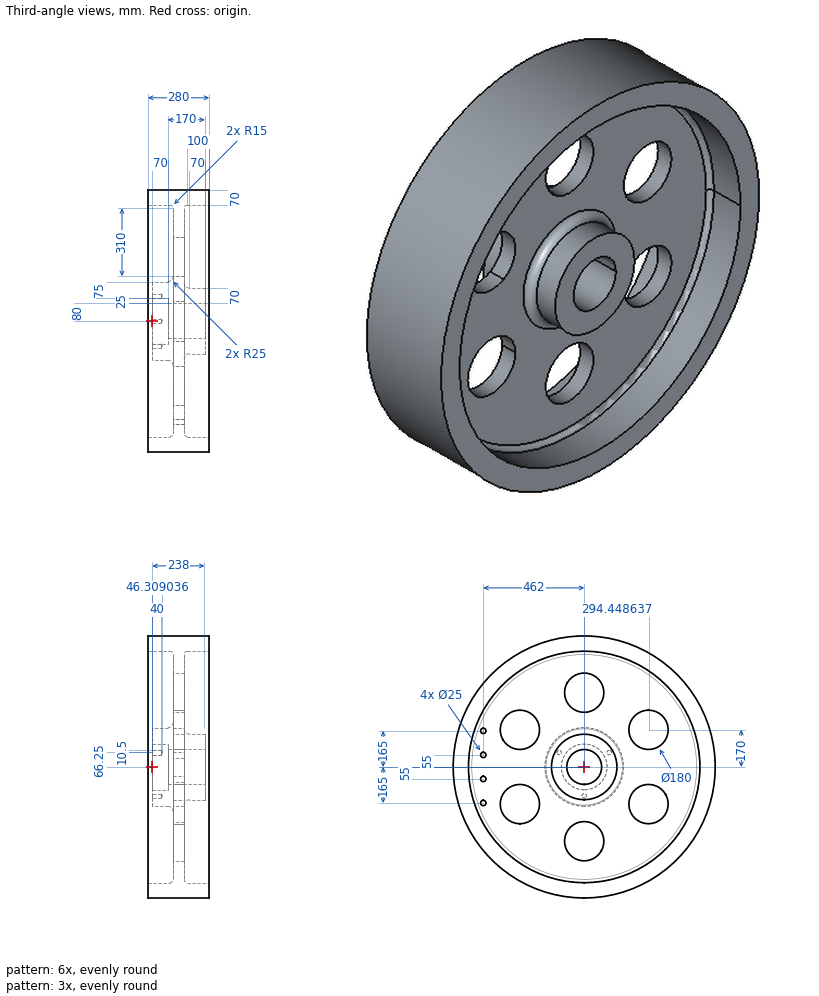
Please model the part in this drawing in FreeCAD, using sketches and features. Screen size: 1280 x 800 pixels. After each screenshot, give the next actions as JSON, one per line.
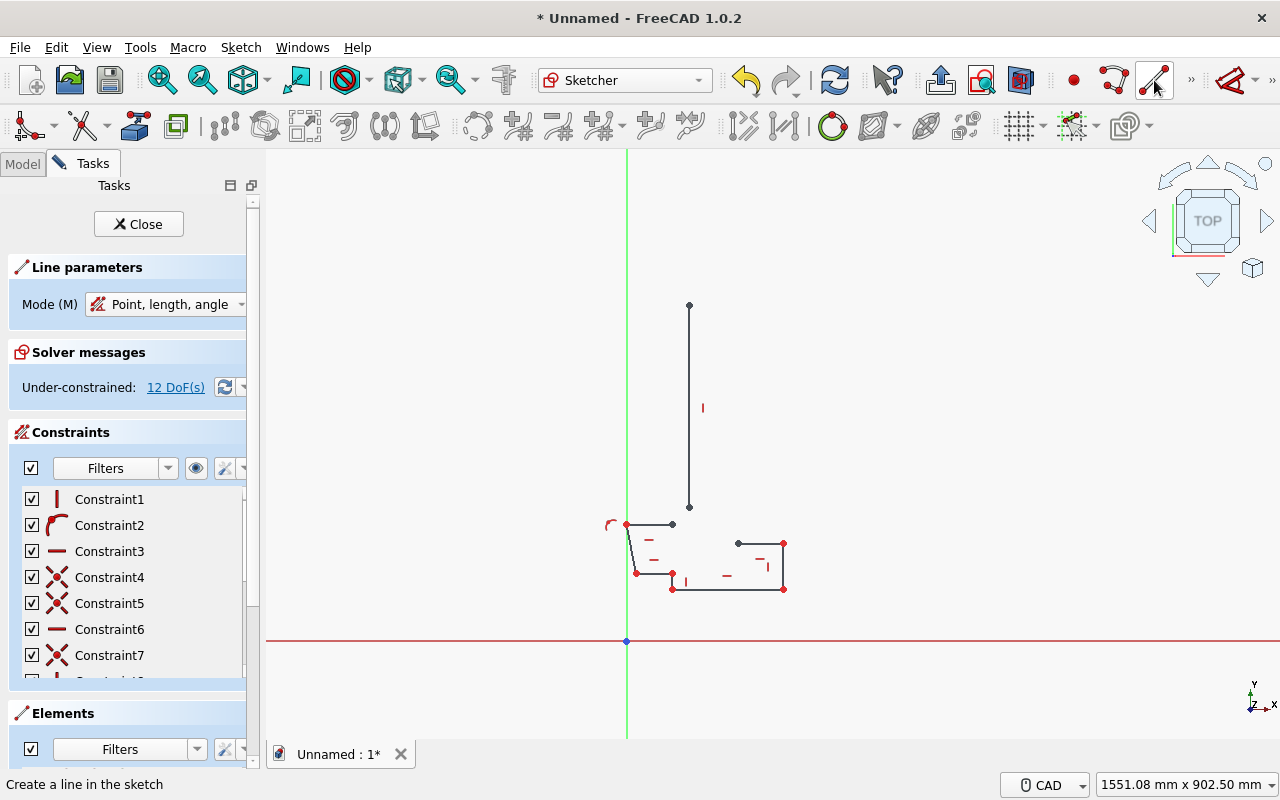
{"action": "left_click", "coordinate": [721, 527]}
{"action": "left_click", "coordinate": [721, 305]}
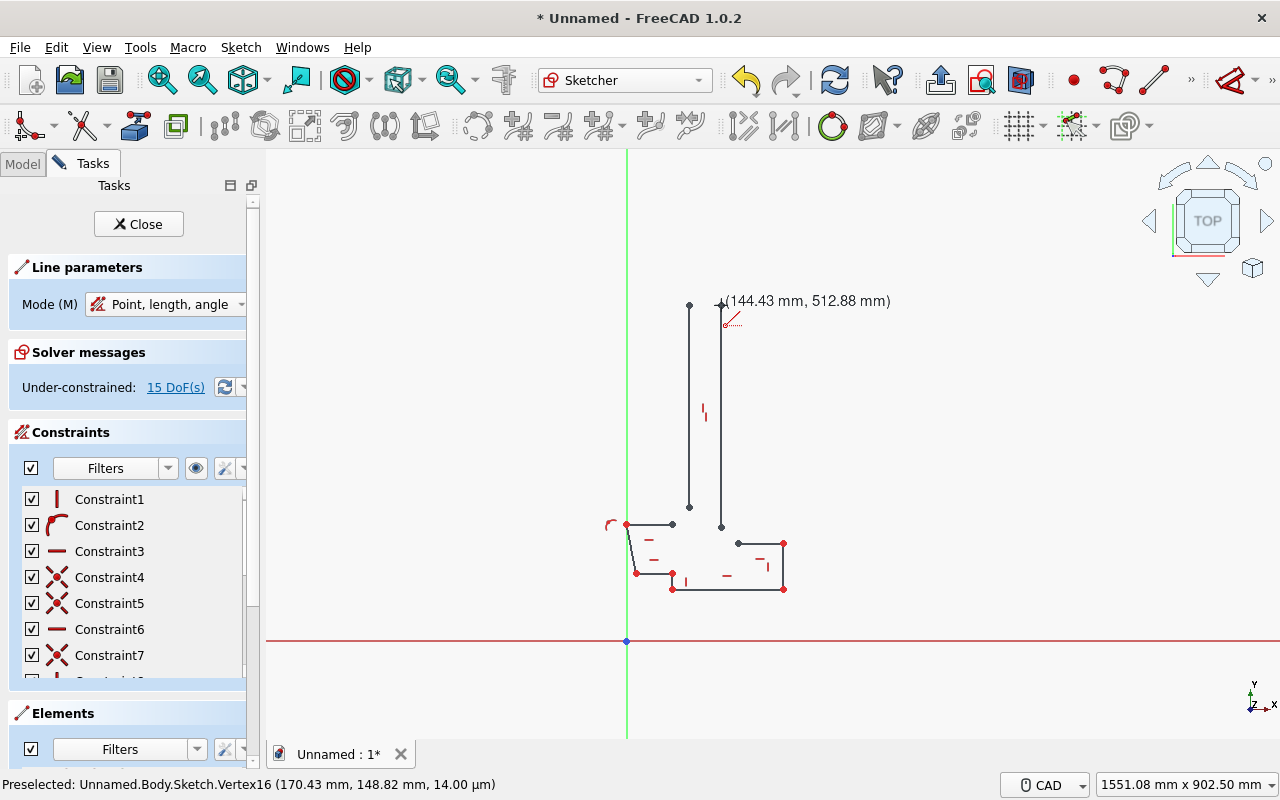
{"action": "key", "text": "g m"}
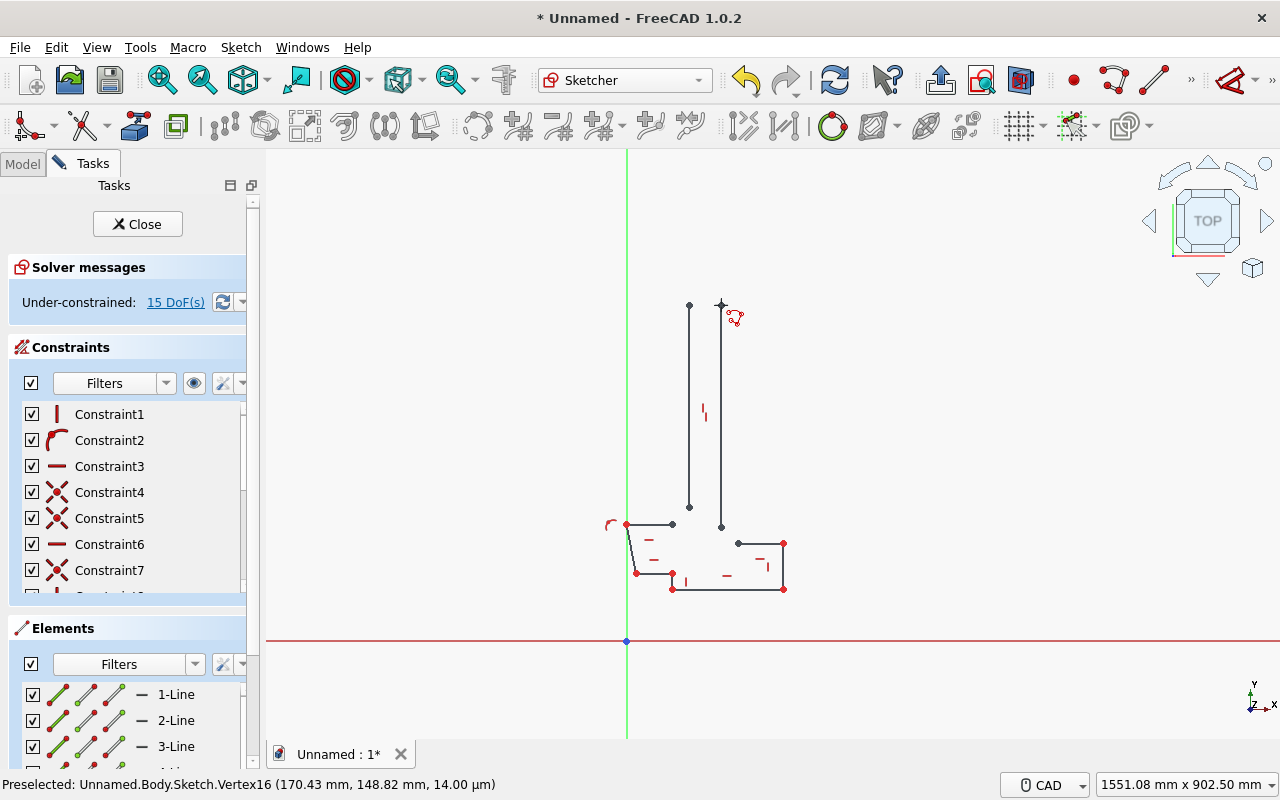
{"action": "left_click", "coordinate": [731, 295]}
{"action": "left_click", "coordinate": [797, 295]}
{"action": "left_click", "coordinate": [797, 249]}
{"action": "left_click", "coordinate": [614, 249]}
{"action": "left_click", "coordinate": [614, 295]}
{"action": "left_click", "coordinate": [679, 295]}
{"action": "right_click", "coordinate": [679, 295]}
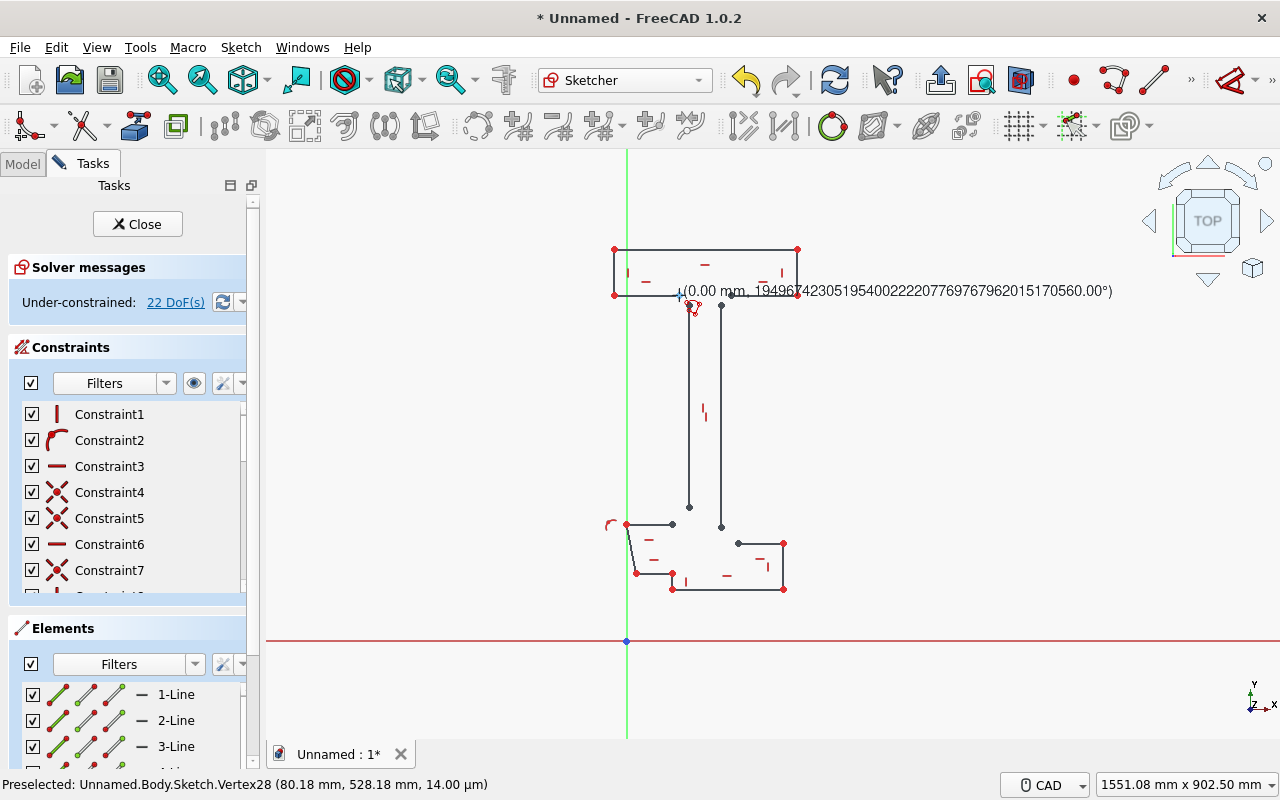
{"action": "key", "text": "g 3 a"}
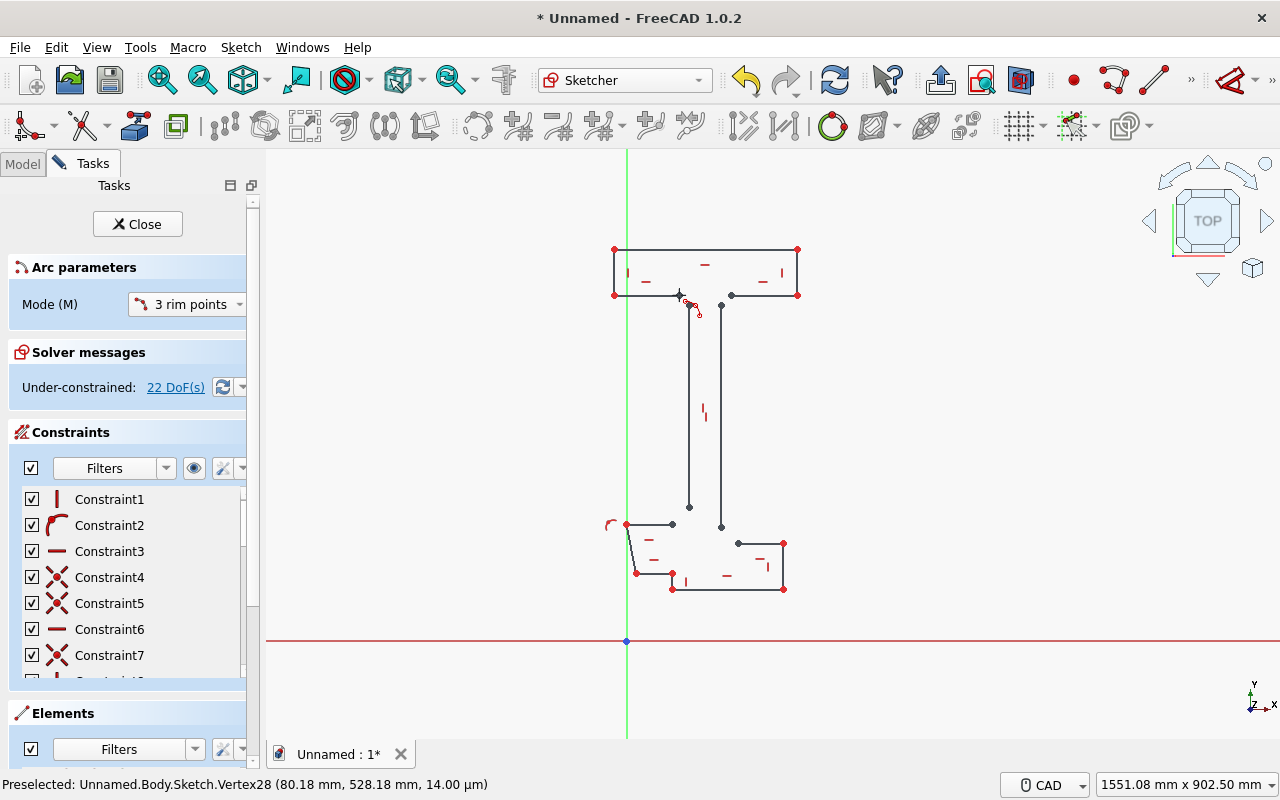
{"action": "left_click", "coordinate": [689, 508]}
{"action": "left_click", "coordinate": [672, 525]}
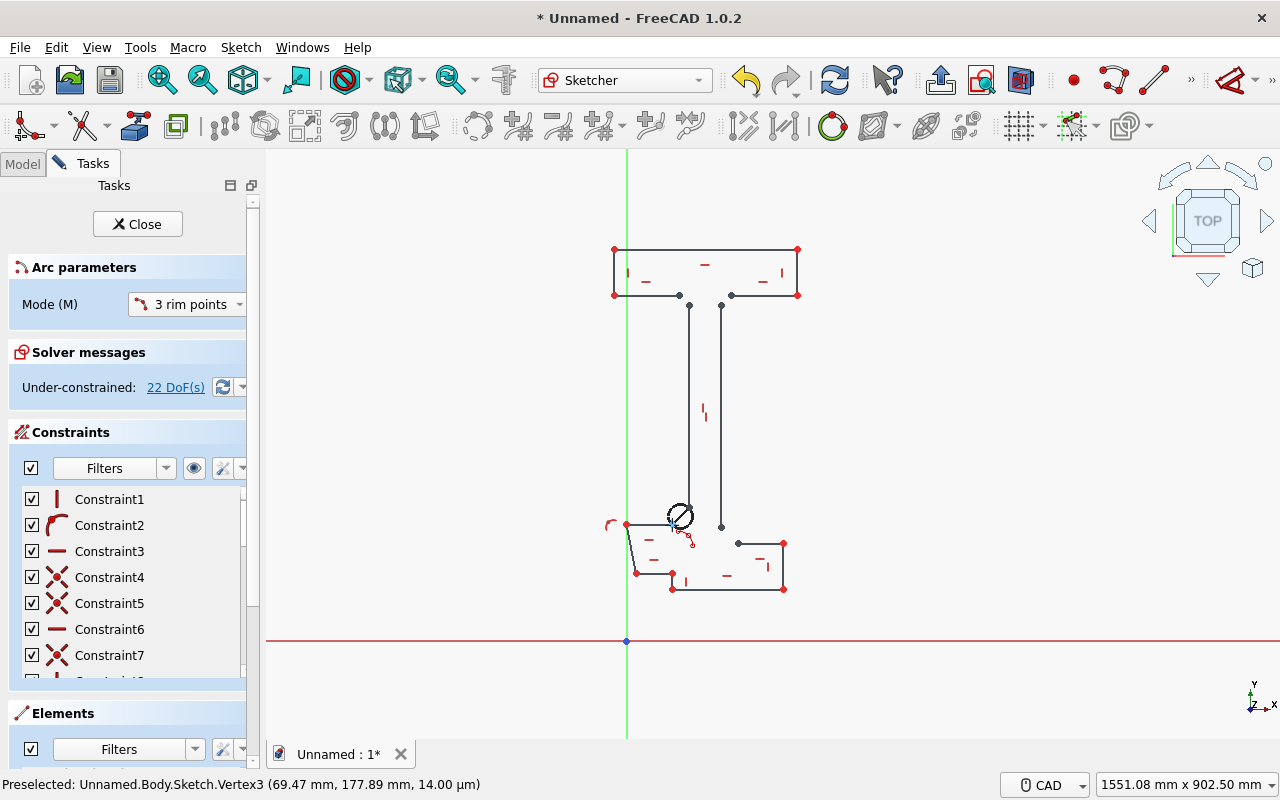
{"action": "scroll", "coordinate": [684, 519], "scroll_direction": "up", "scroll_amount": 6}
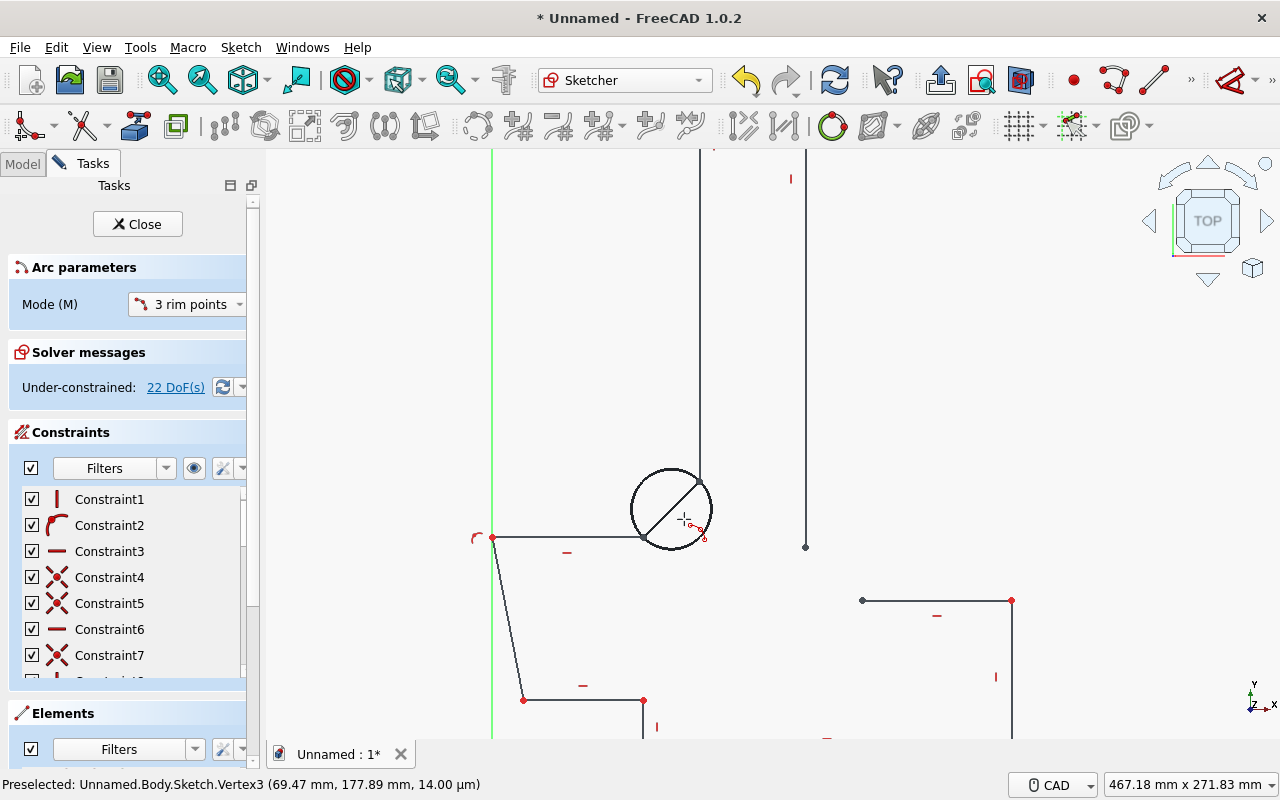
{"action": "left_click", "coordinate": [683, 517]}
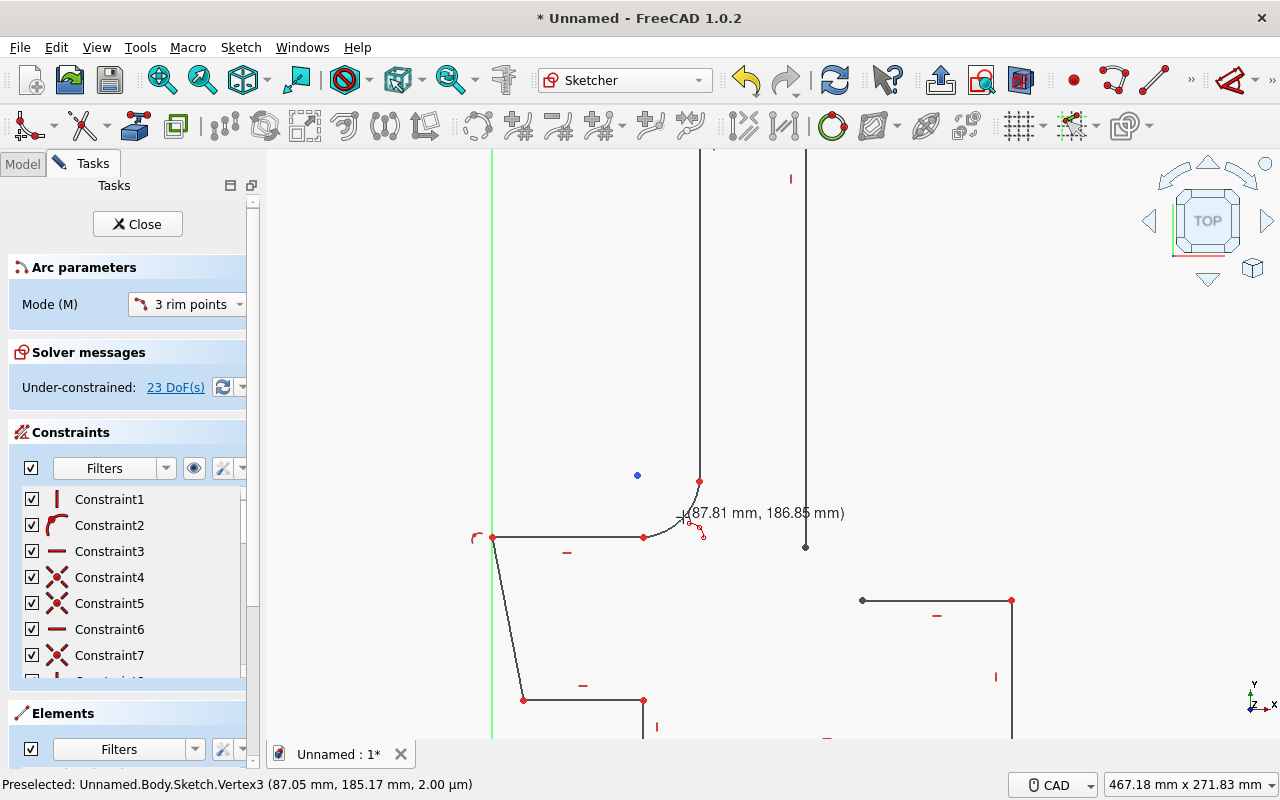
{"action": "left_click", "coordinate": [862, 601]}
{"action": "left_click", "coordinate": [806, 547]}
{"action": "left_click", "coordinate": [823, 582]}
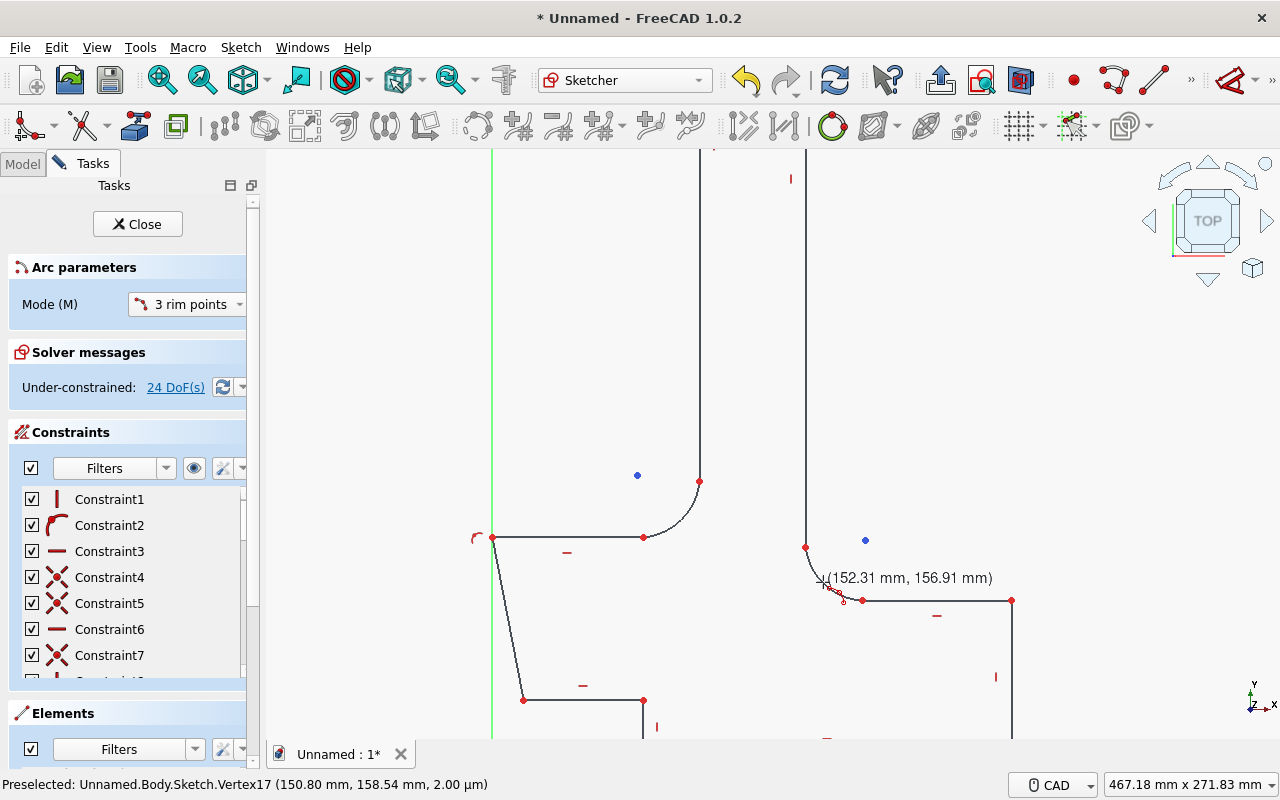
{"action": "scroll", "coordinate": [684, 518], "scroll_direction": "down", "scroll_amount": 6}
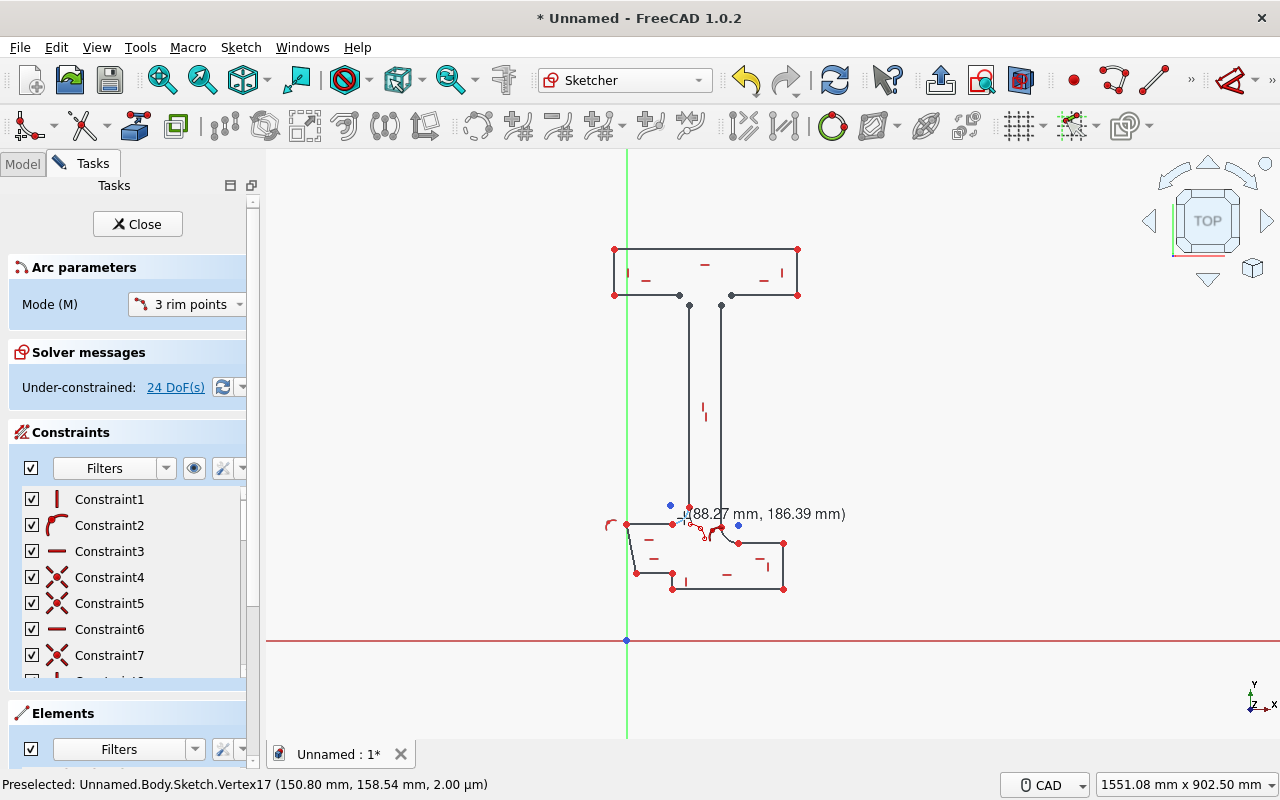
{"action": "left_click", "coordinate": [721, 305]}
{"action": "left_click", "coordinate": [731, 295]}